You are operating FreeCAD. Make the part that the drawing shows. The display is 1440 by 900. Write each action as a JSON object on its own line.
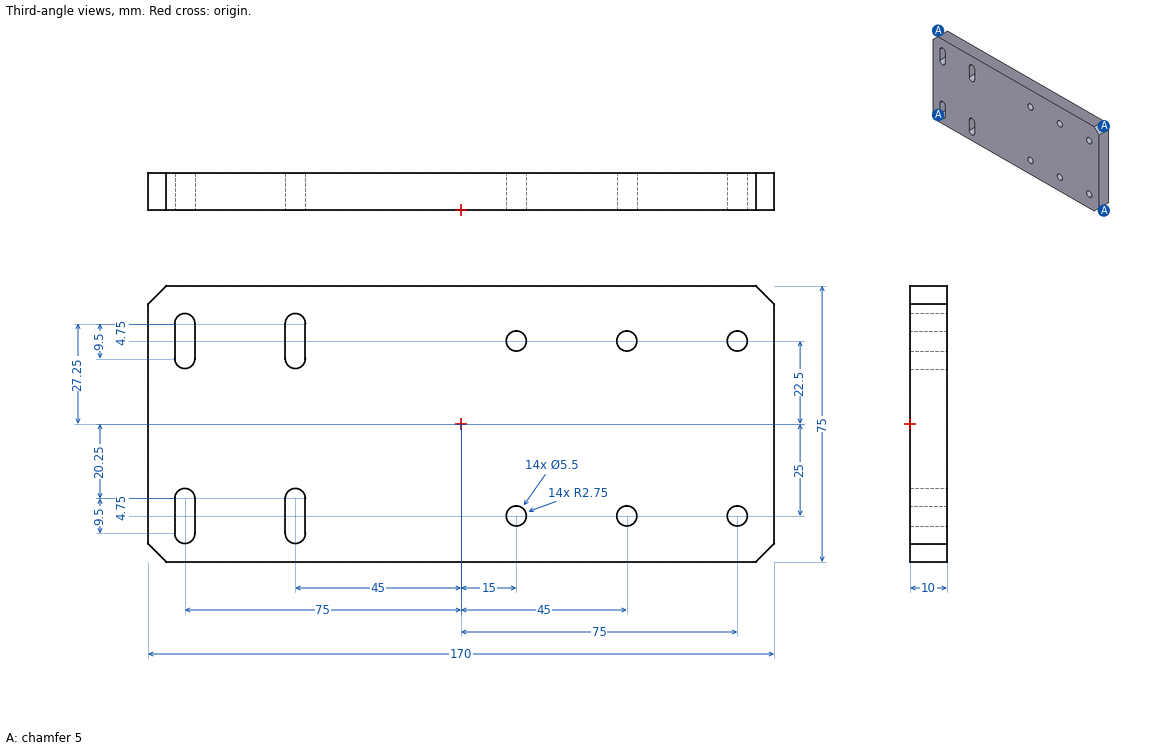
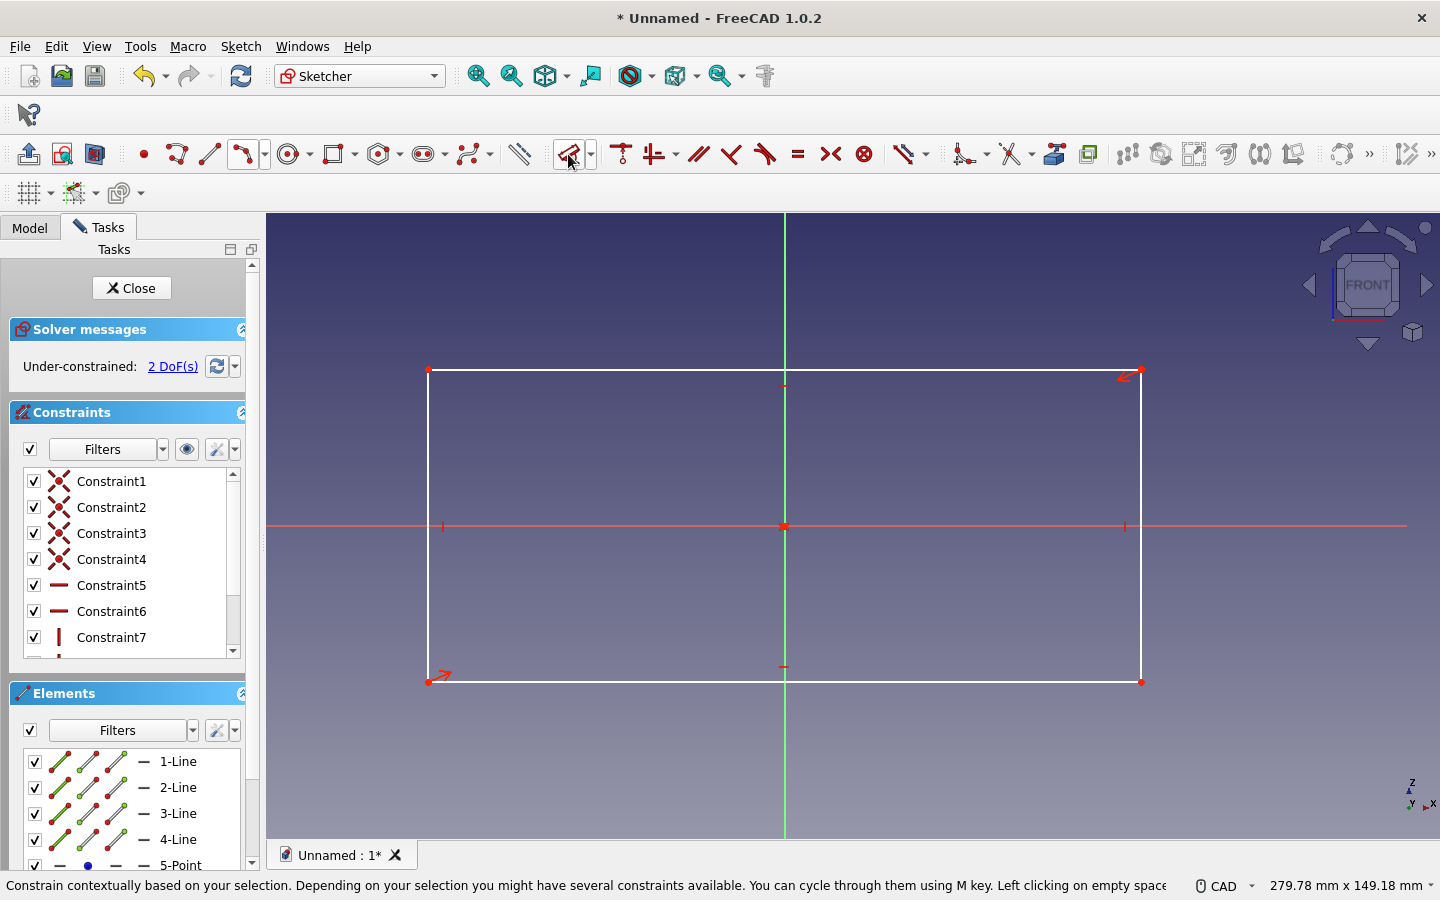
{"action": "left_click", "coordinate": [1141, 589]}
{"action": "left_click", "coordinate": [1175, 454]}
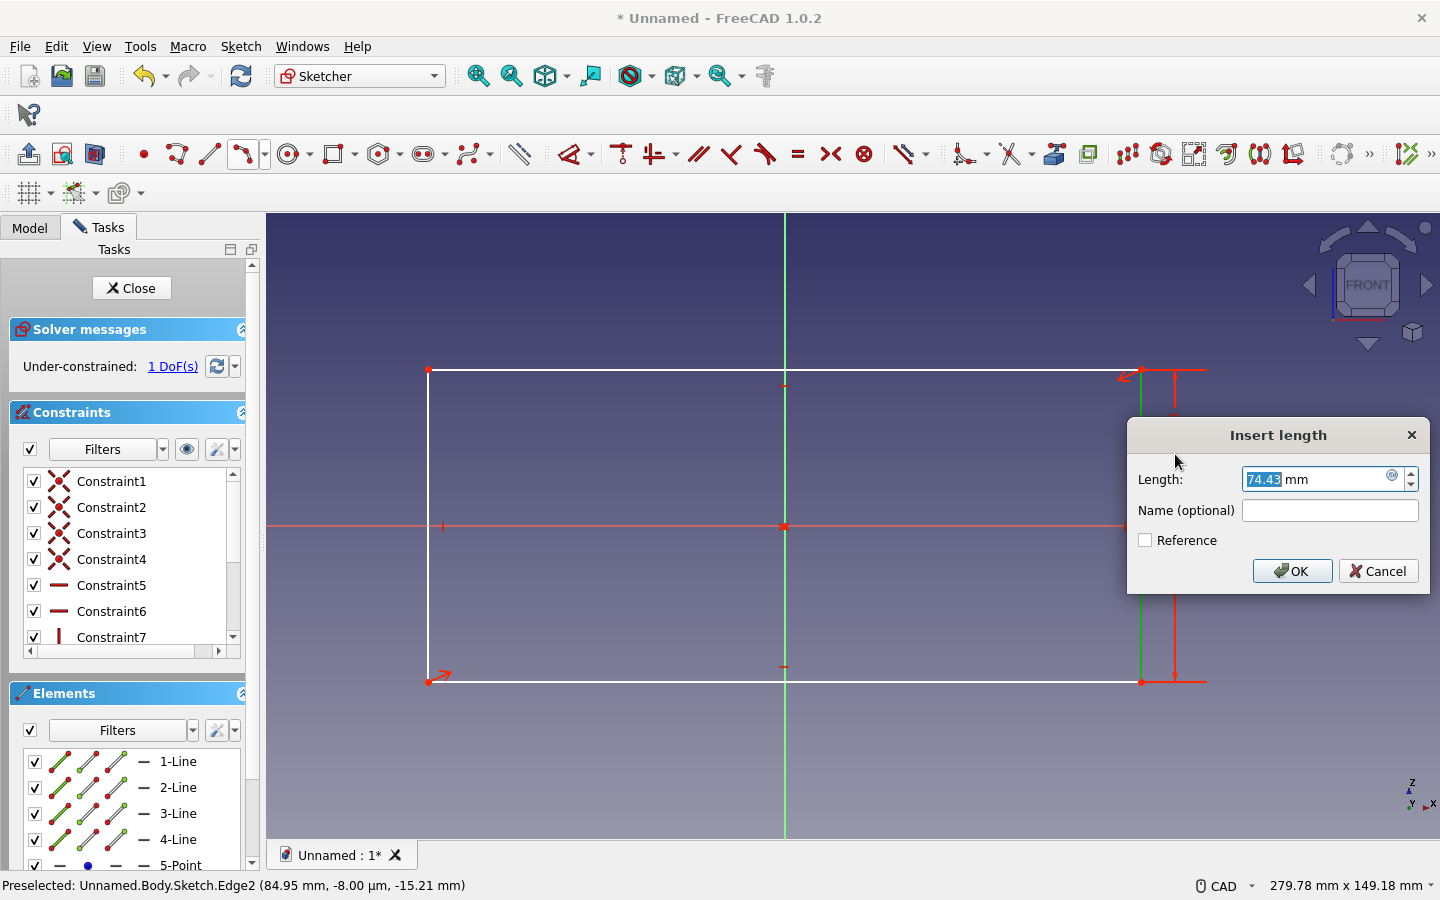
{"action": "type", "text": "75"}
{"action": "key", "text": "Return"}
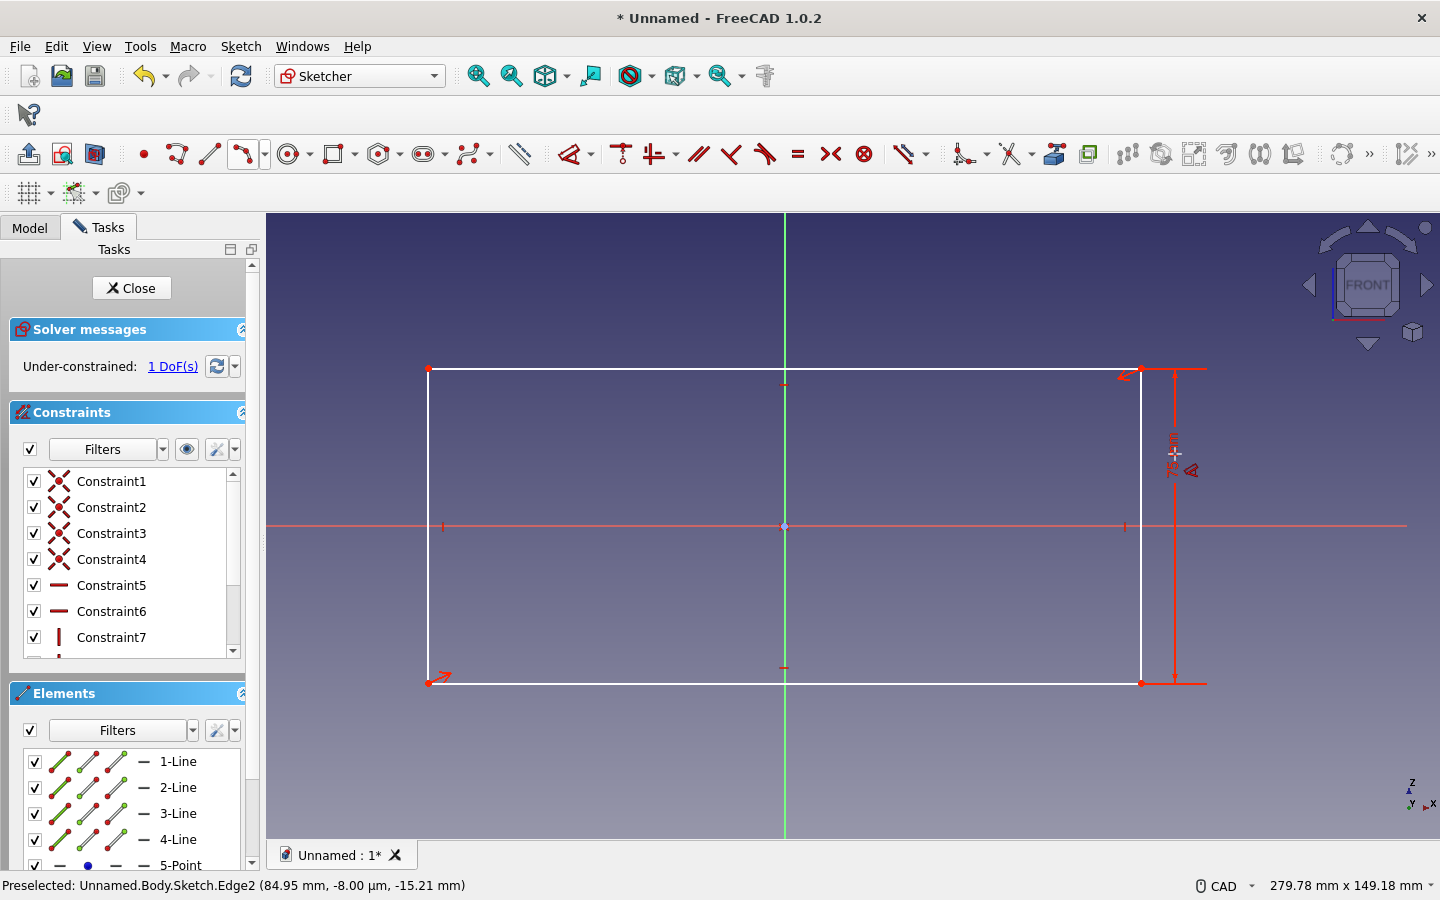
{"action": "left_click", "coordinate": [642, 684]}
{"action": "left_click", "coordinate": [621, 718]}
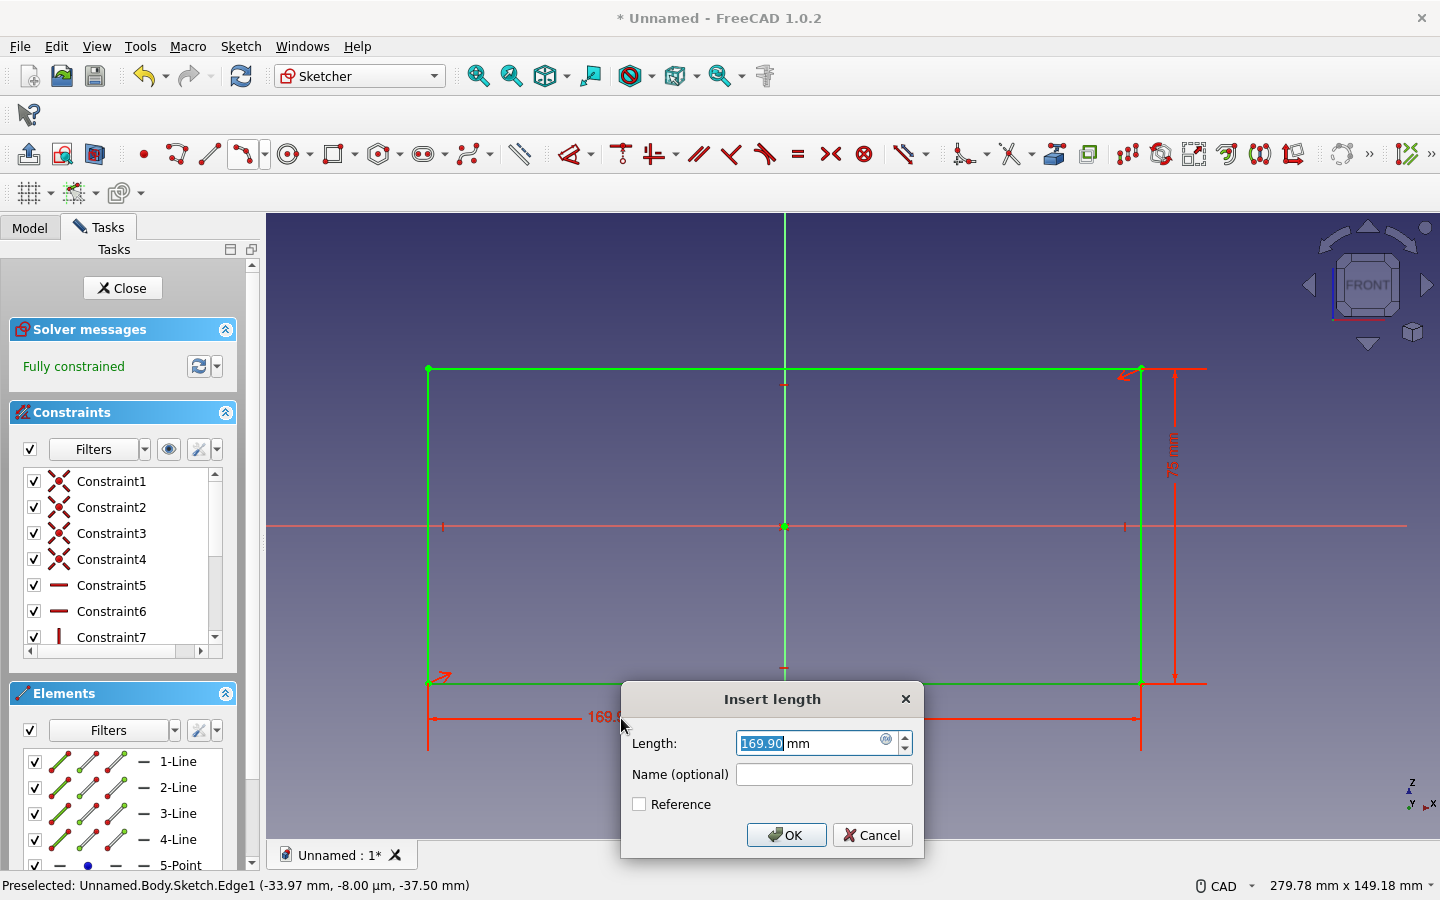
{"action": "type", "text": "170"}
{"action": "key", "text": "Return"}
{"action": "key", "text": "Escape"}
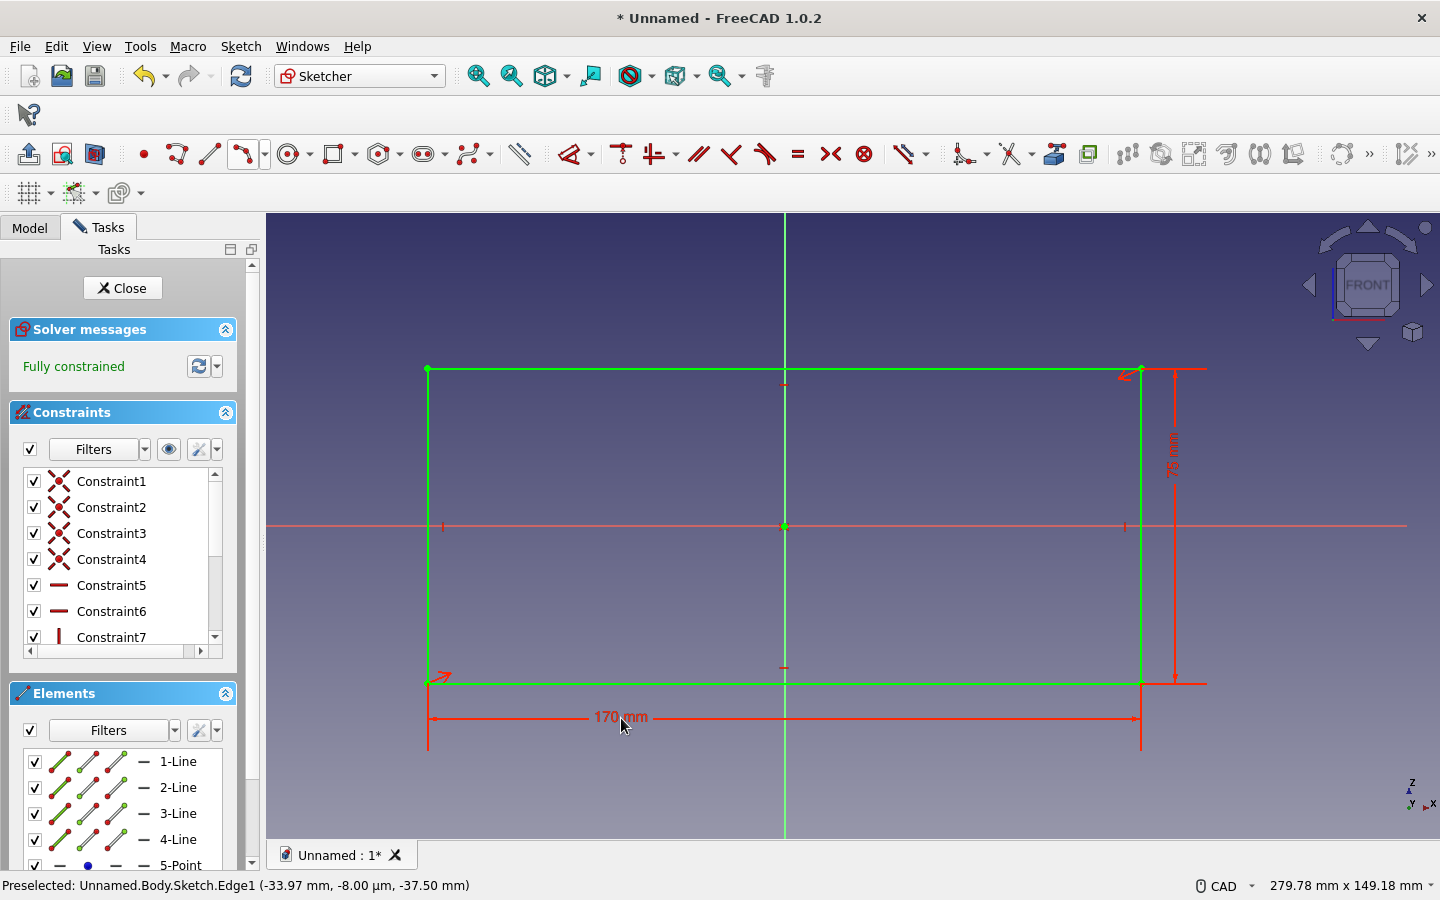
{"action": "left_click", "coordinate": [123, 288]}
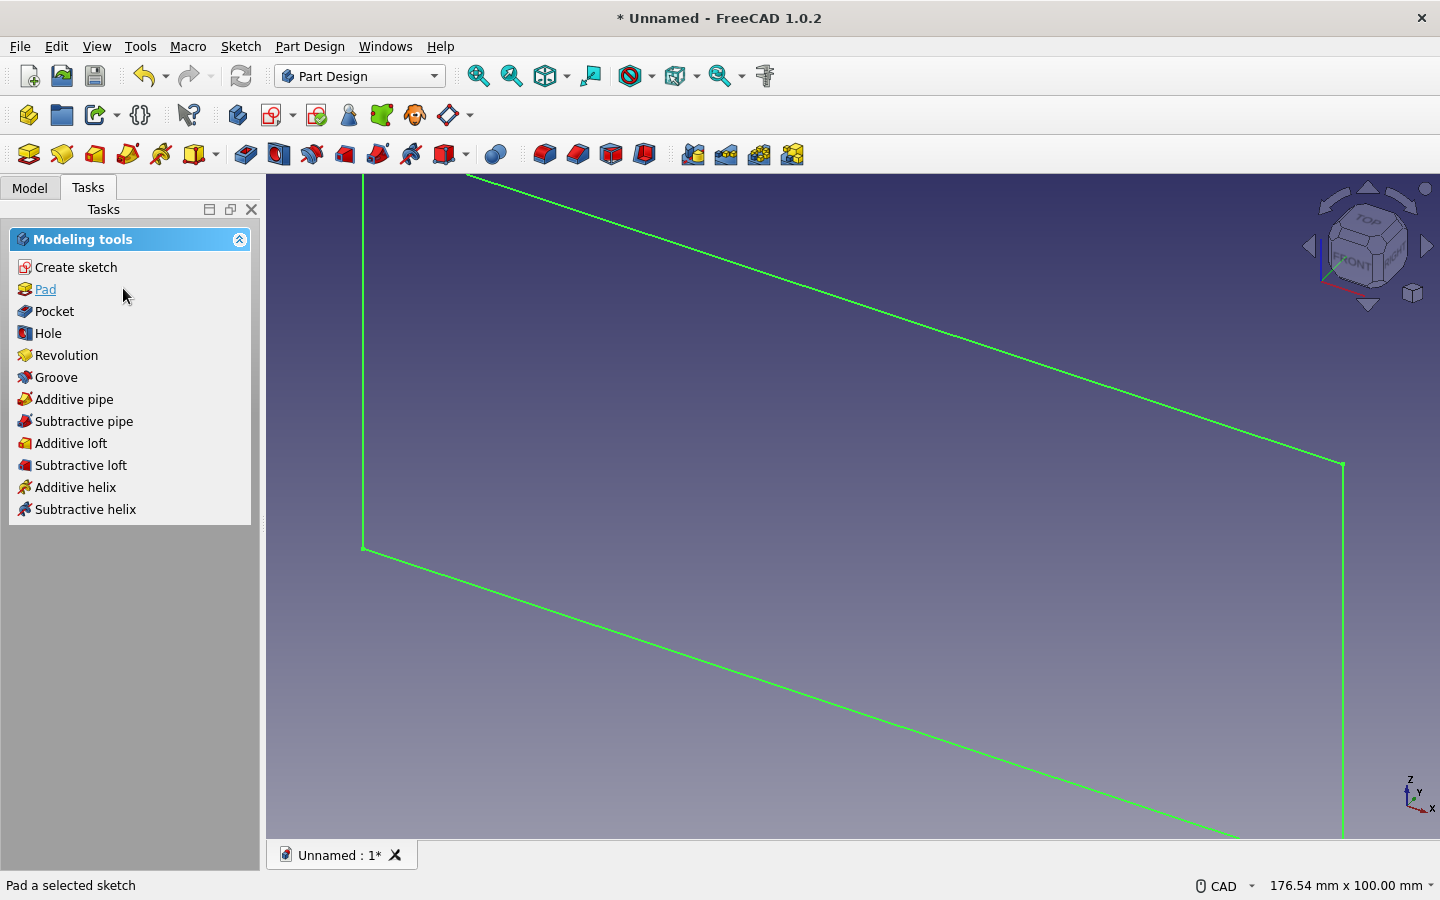
{"action": "left_click", "coordinate": [29, 154]}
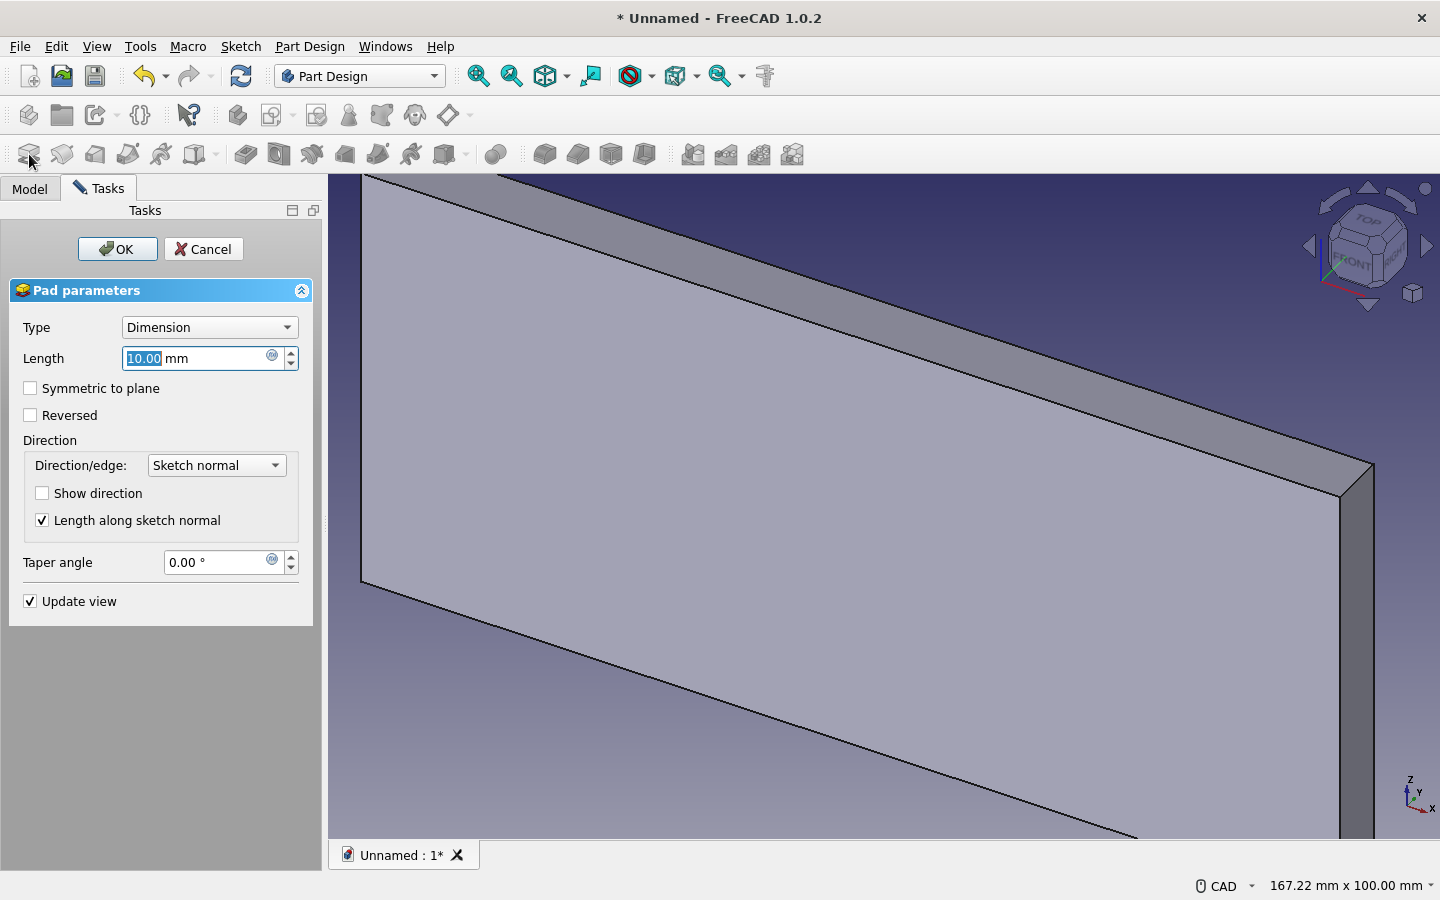
{"action": "type", "text": "10"}
{"action": "key", "text": "Tab"}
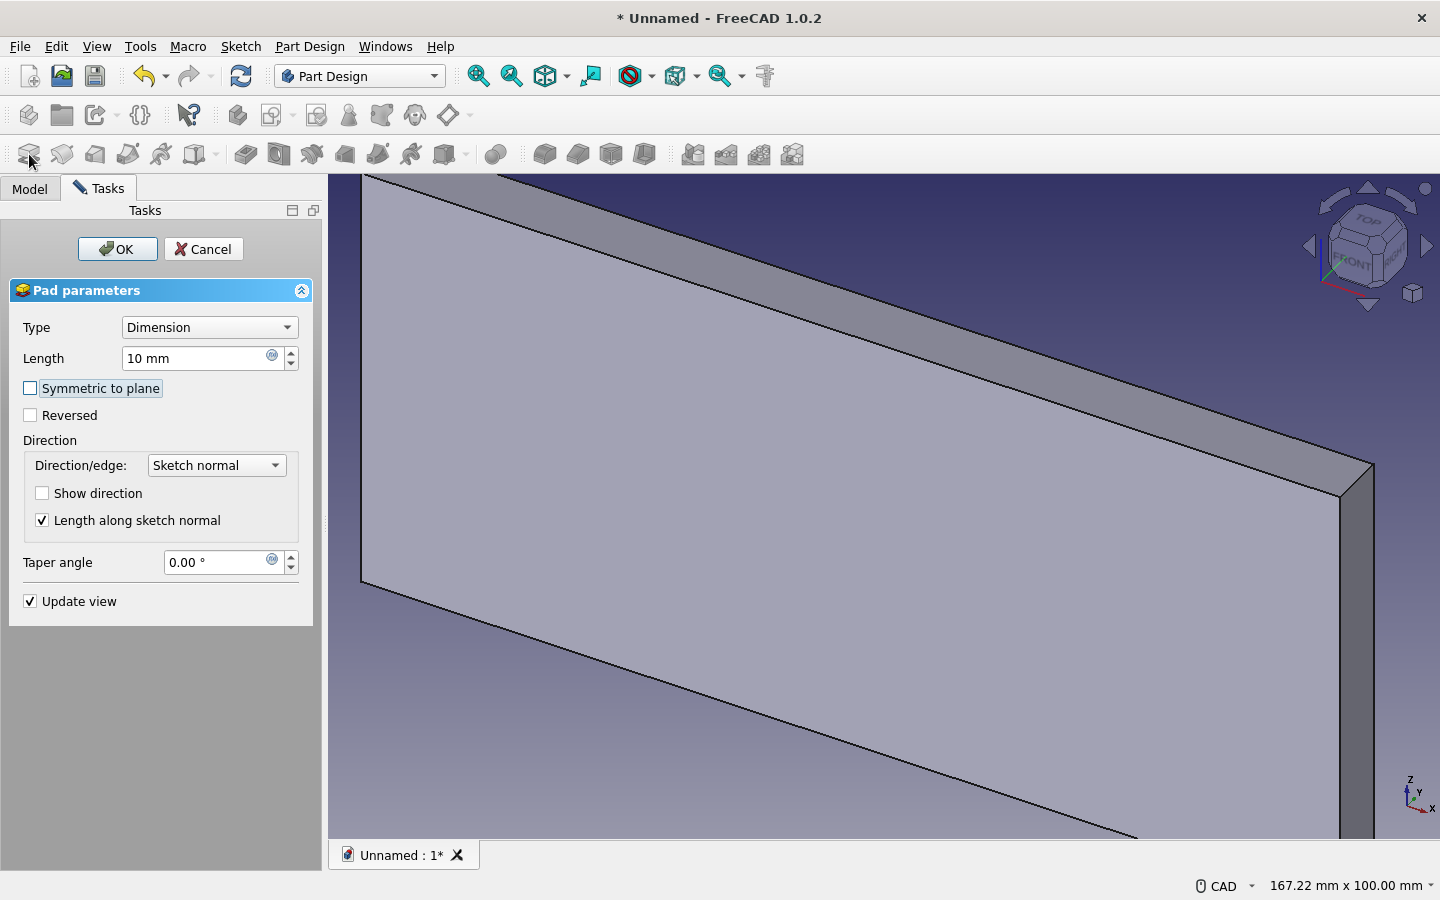
{"action": "left_click", "coordinate": [31, 415]}